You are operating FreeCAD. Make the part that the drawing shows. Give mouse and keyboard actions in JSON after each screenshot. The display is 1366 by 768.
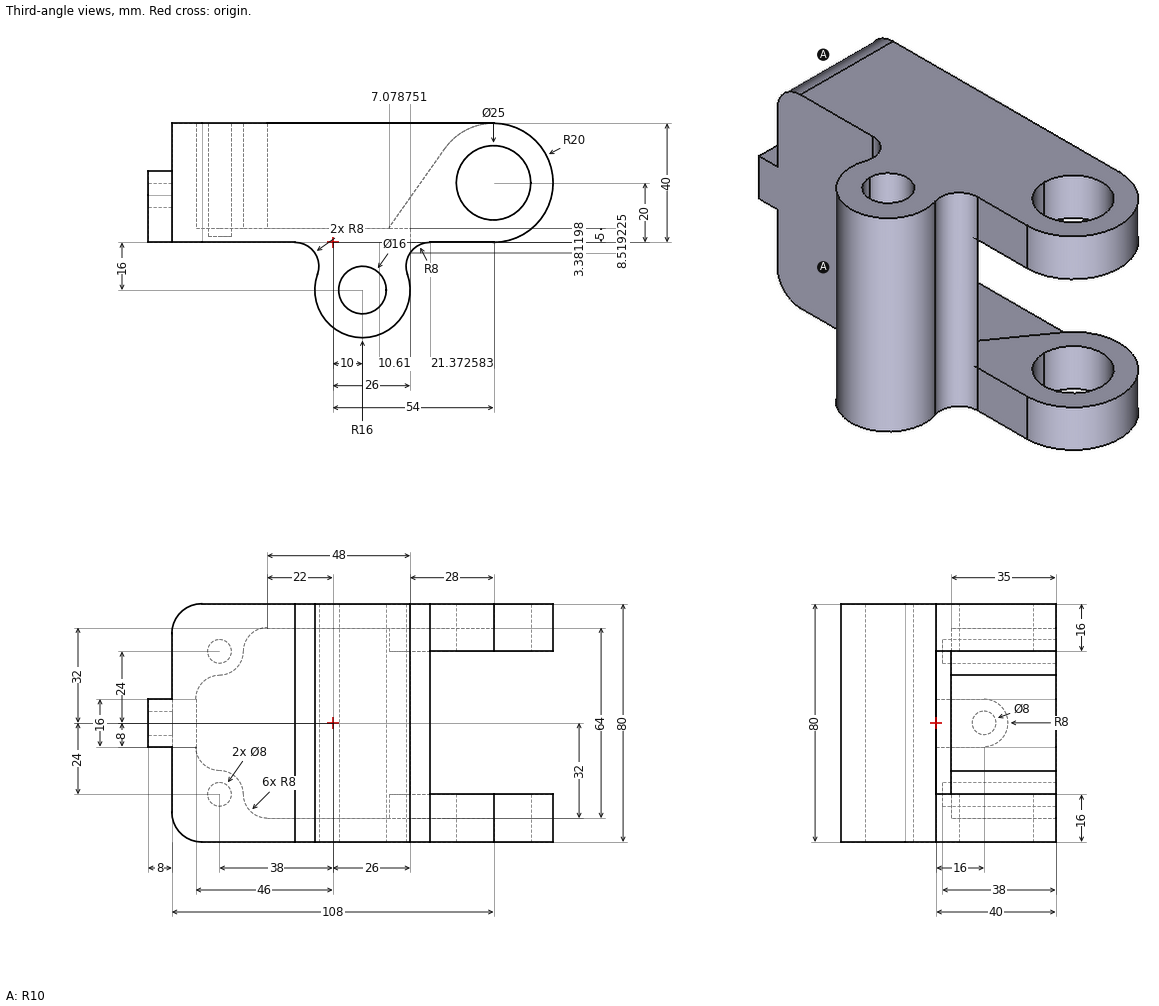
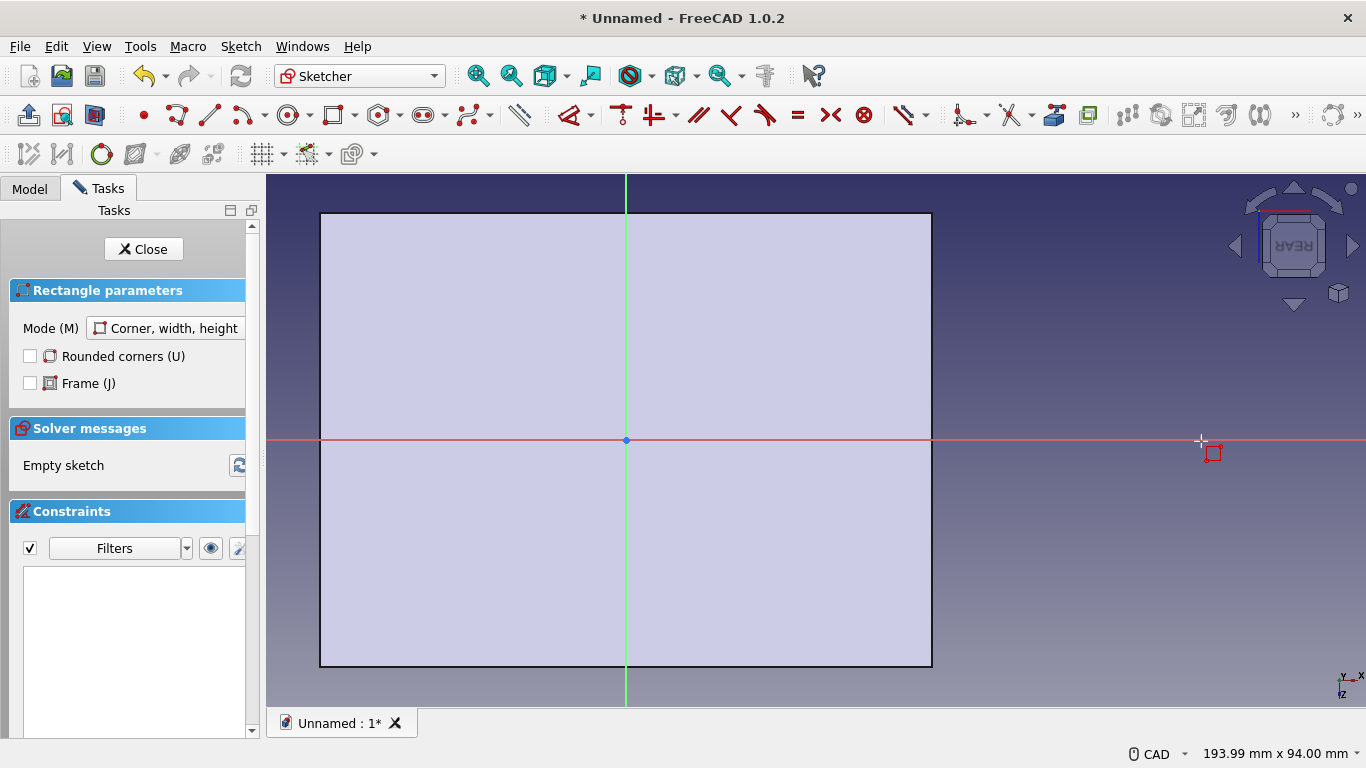
{"action": "left_click", "coordinate": [774, 259]}
{"action": "mouse_move", "coordinate": [932, 621]}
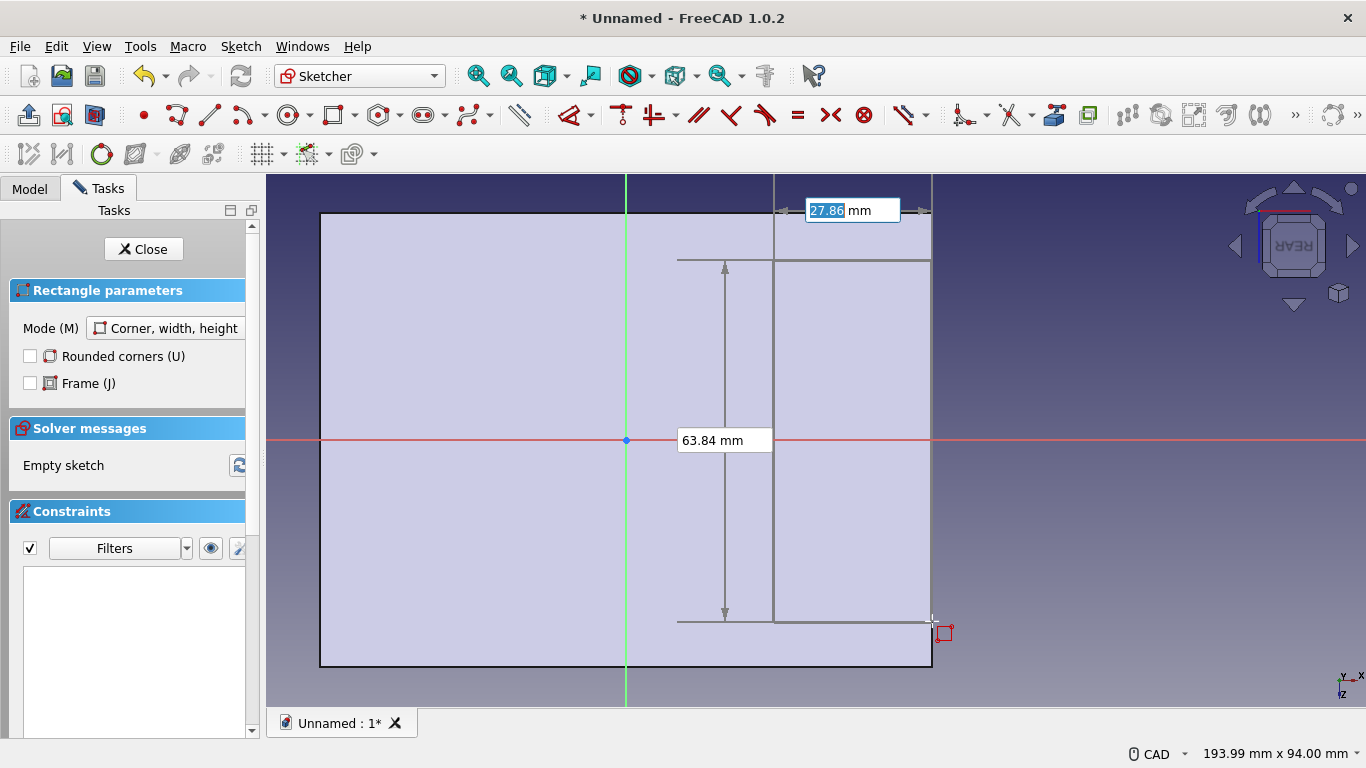
{"action": "type", "text": "28"}
{"action": "key", "text": "Tab"}
{"action": "type", "text": "64"}
{"action": "key", "text": "Return"}
{"action": "key", "text": "Escape"}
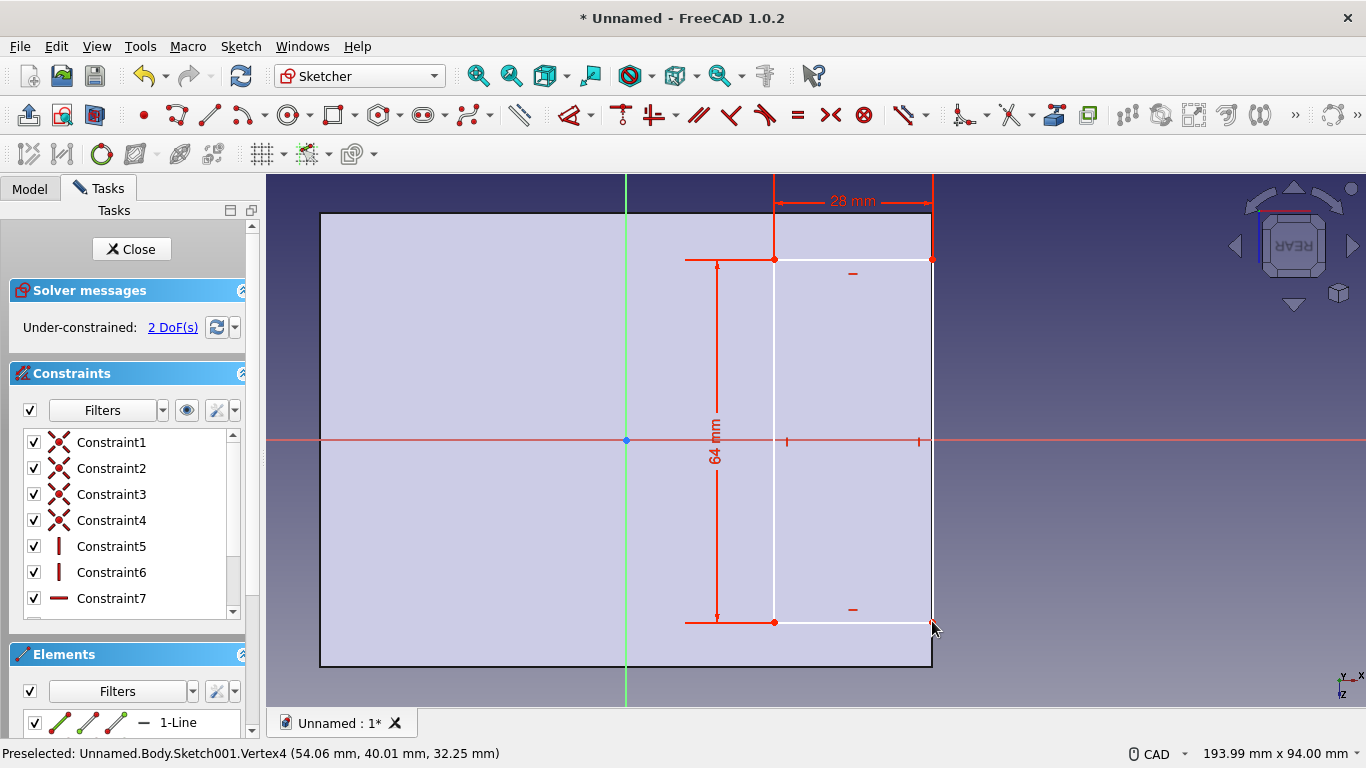
{"action": "left_click", "coordinate": [568, 116]}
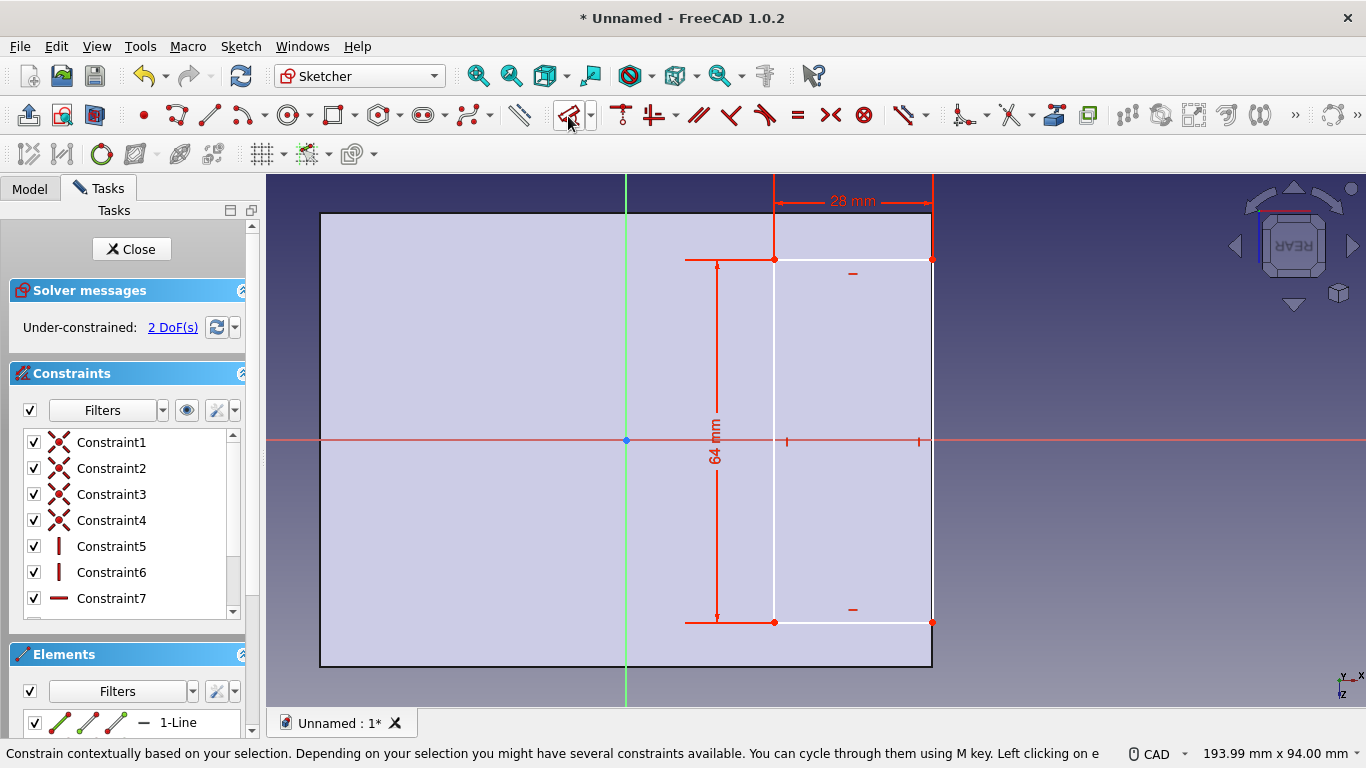
{"action": "left_click", "coordinate": [774, 260]}
{"action": "left_click", "coordinate": [700, 226]}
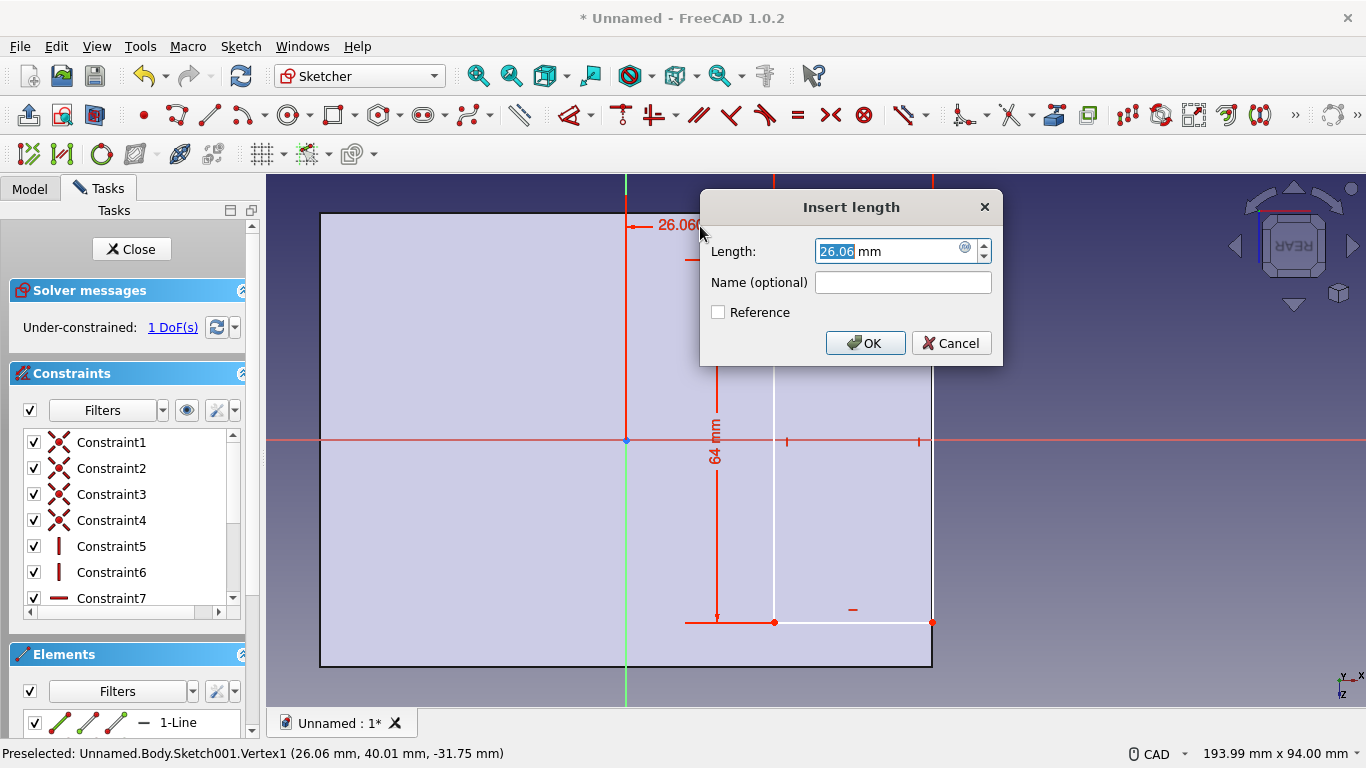
{"action": "type", "text": "26"}
{"action": "key", "text": "Return"}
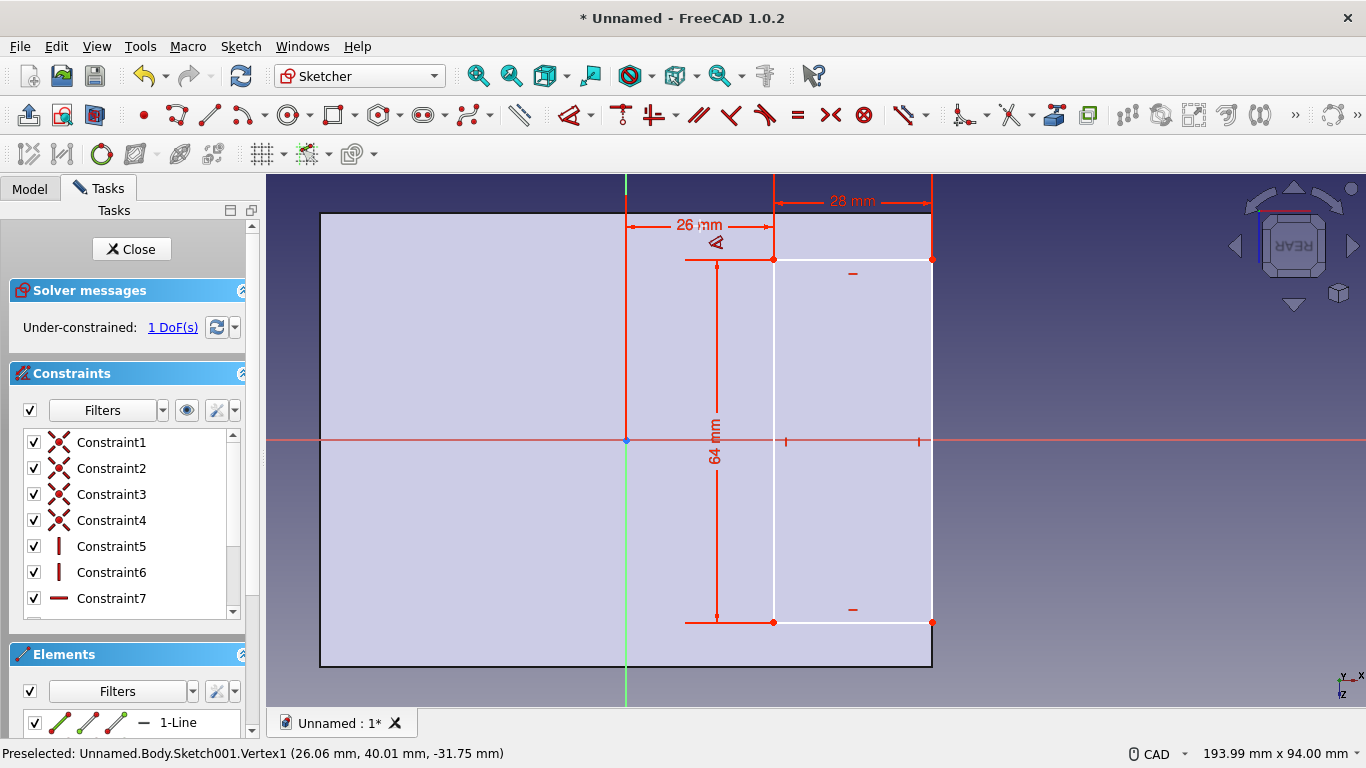
{"action": "left_click", "coordinate": [774, 260]}
{"action": "left_click", "coordinate": [592, 350]}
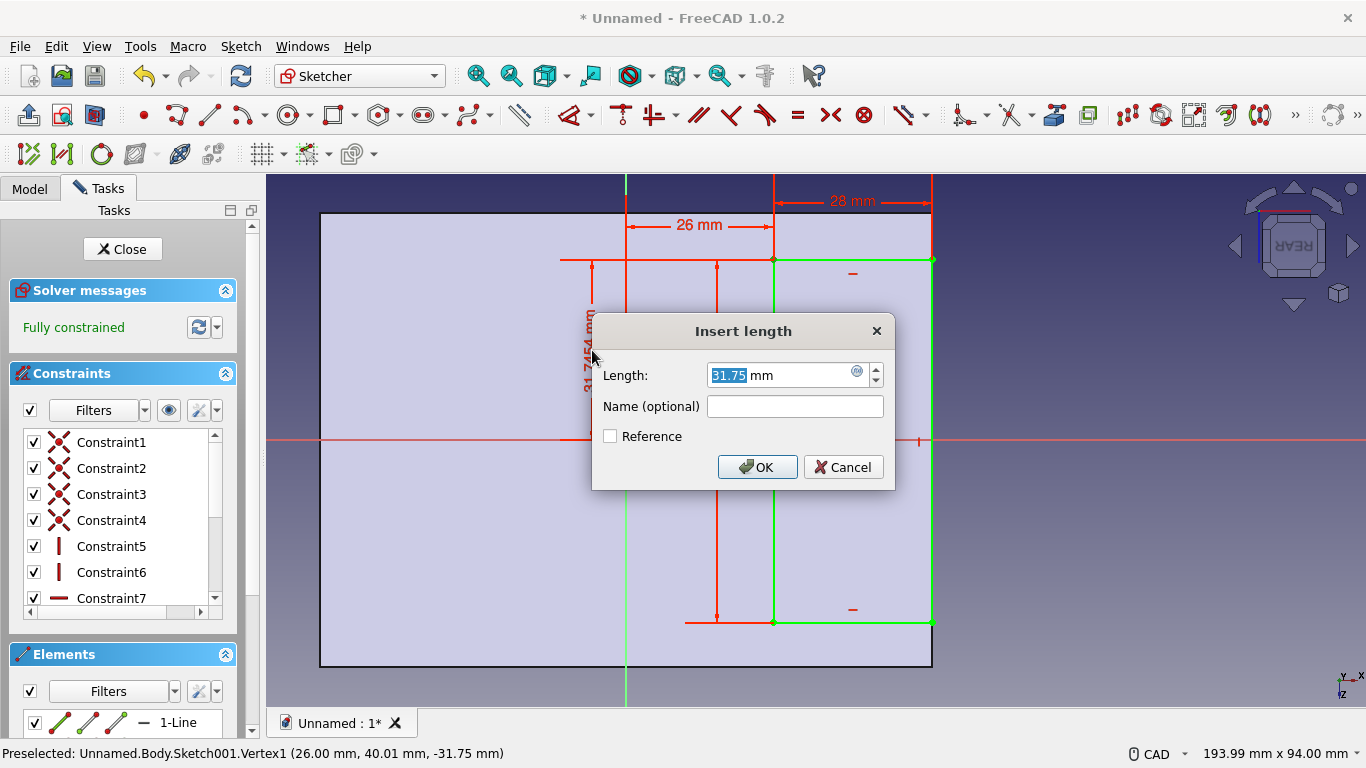
{"action": "type", "text": "32"}
{"action": "key", "text": "Return"}
{"action": "key", "text": "Escape"}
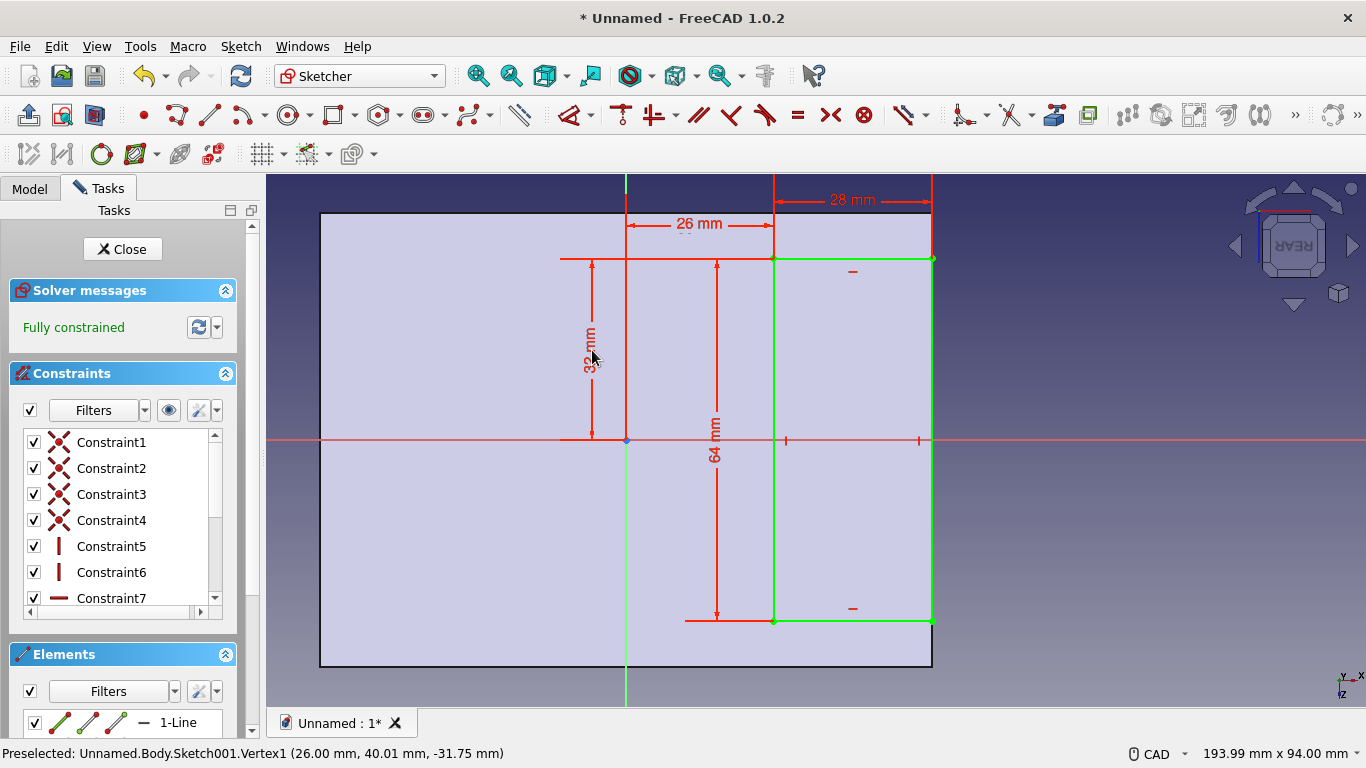
{"action": "left_click", "coordinate": [123, 249]}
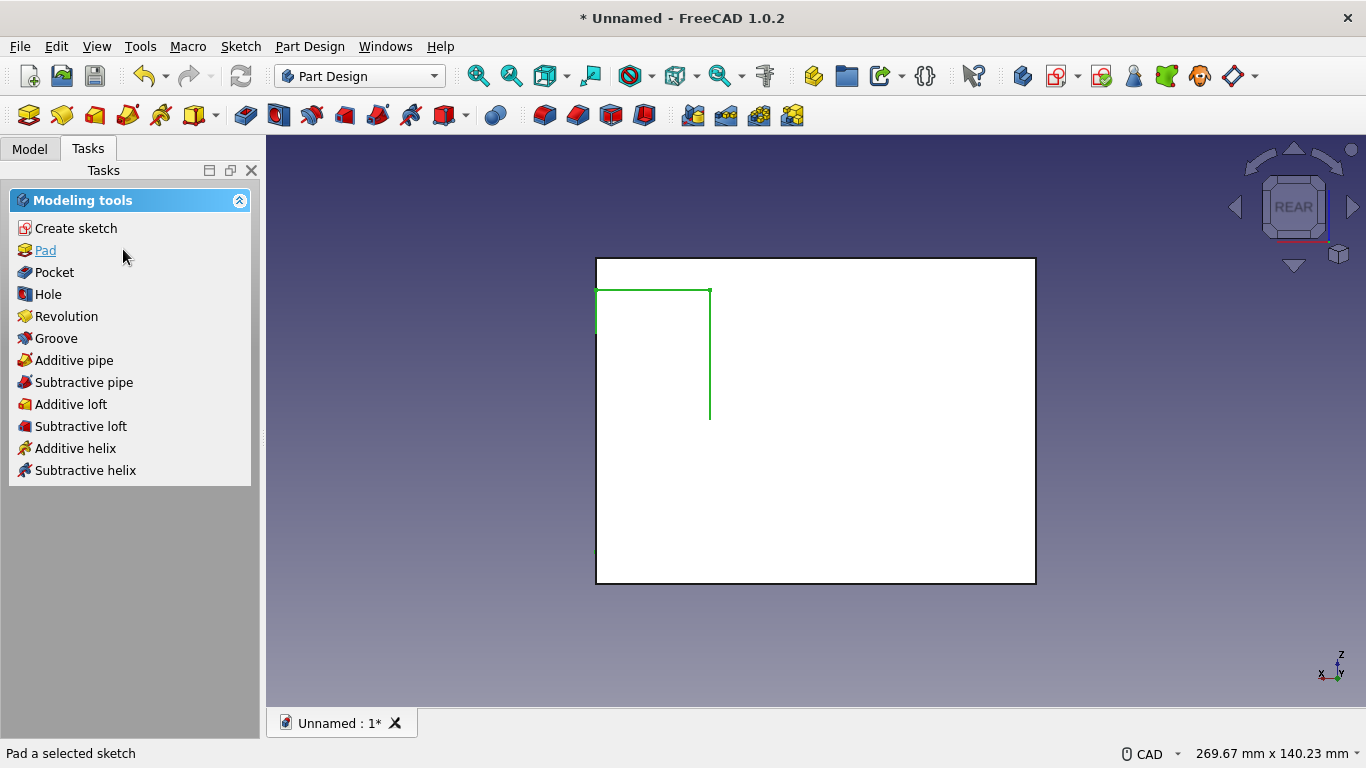
{"action": "left_click", "coordinate": [246, 116]}